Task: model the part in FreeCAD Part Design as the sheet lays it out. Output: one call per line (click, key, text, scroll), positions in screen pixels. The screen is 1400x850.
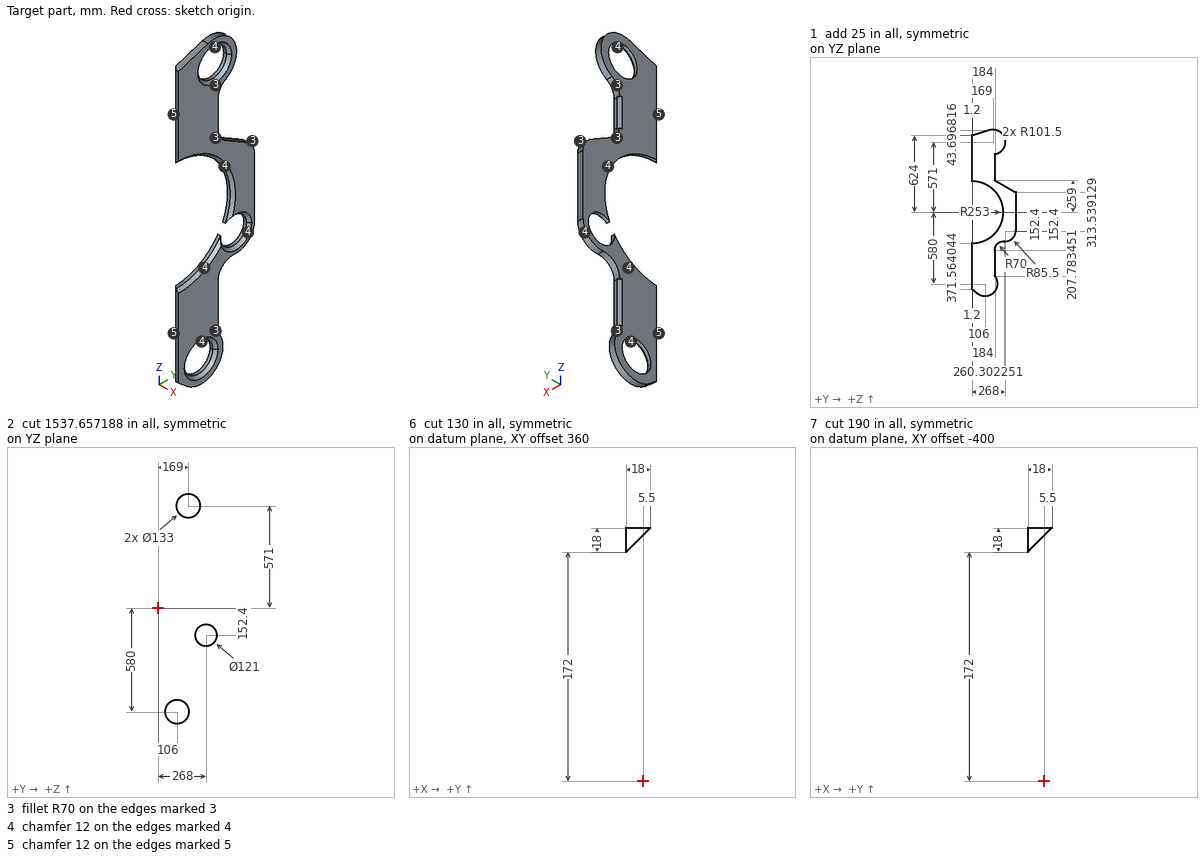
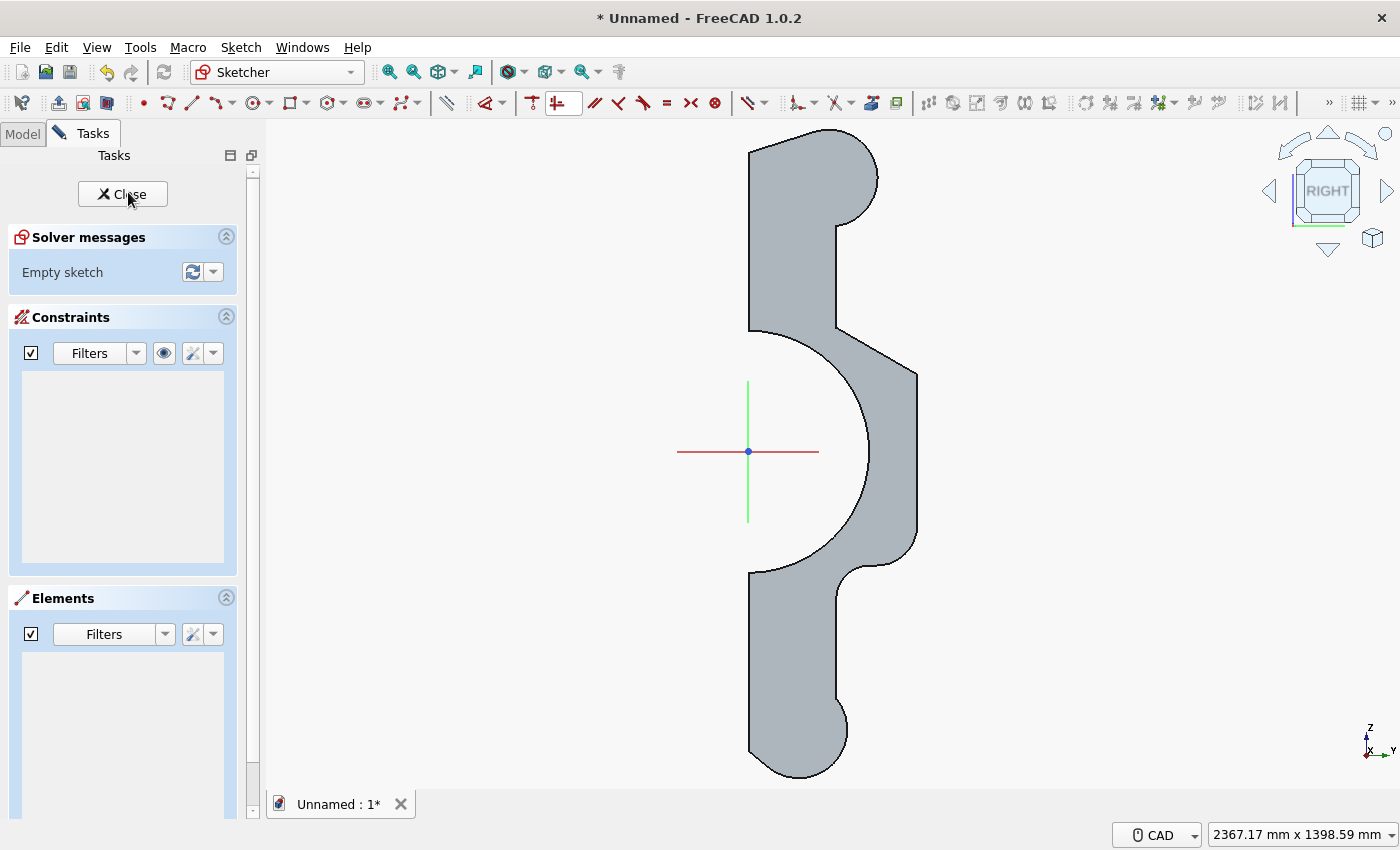
key(q)
key(s)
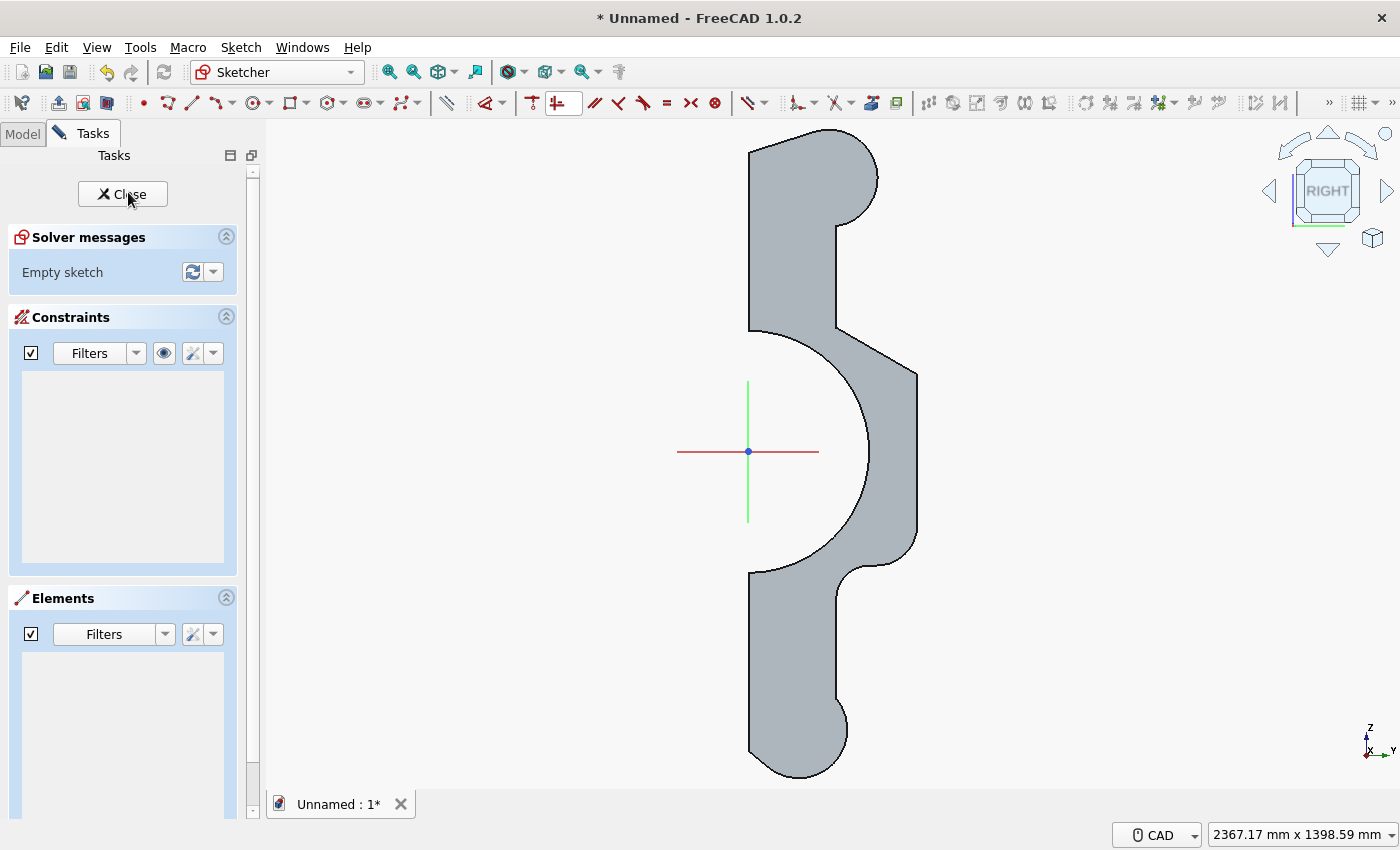
scroll(638, 454, down, 2)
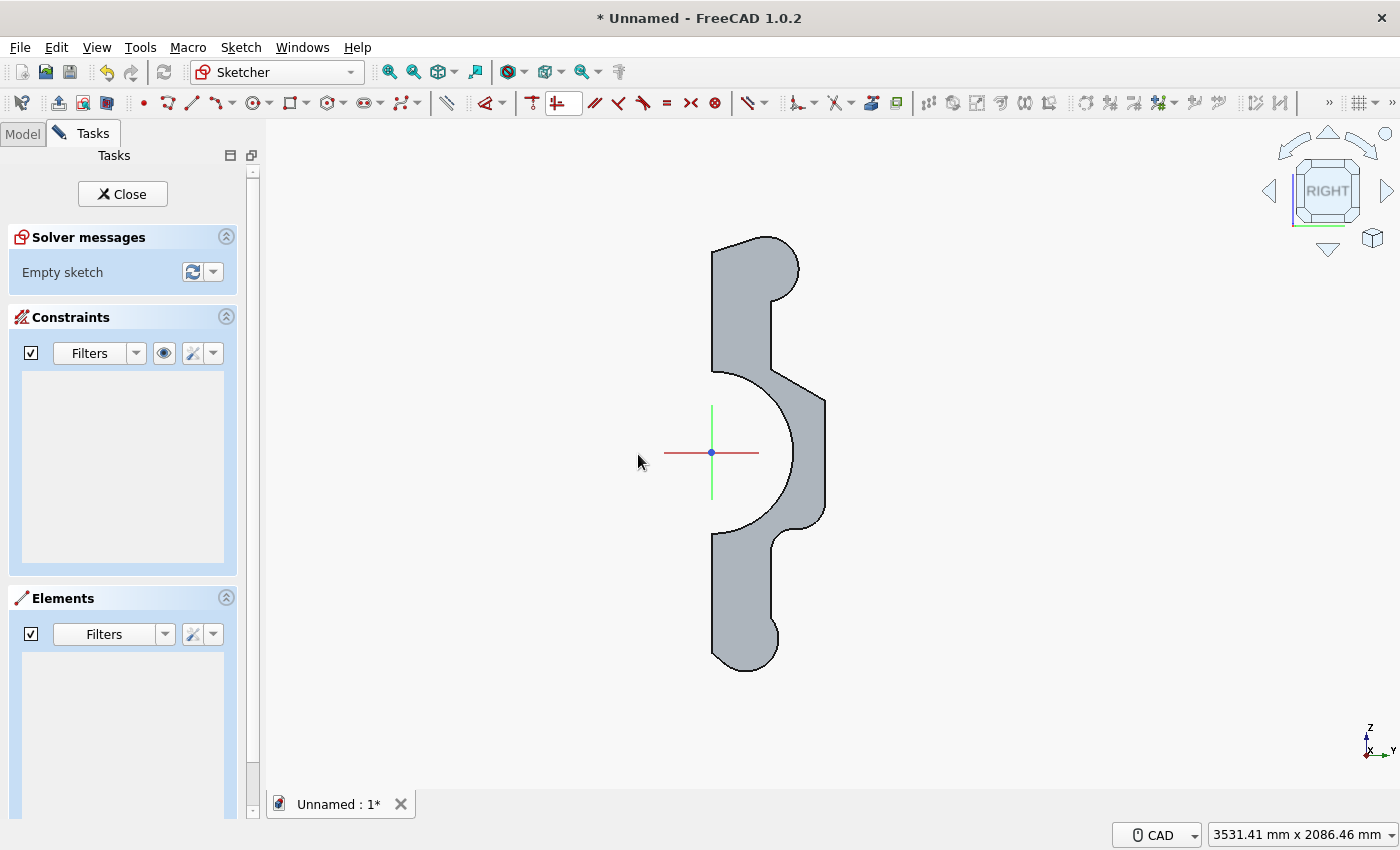
click(254, 104)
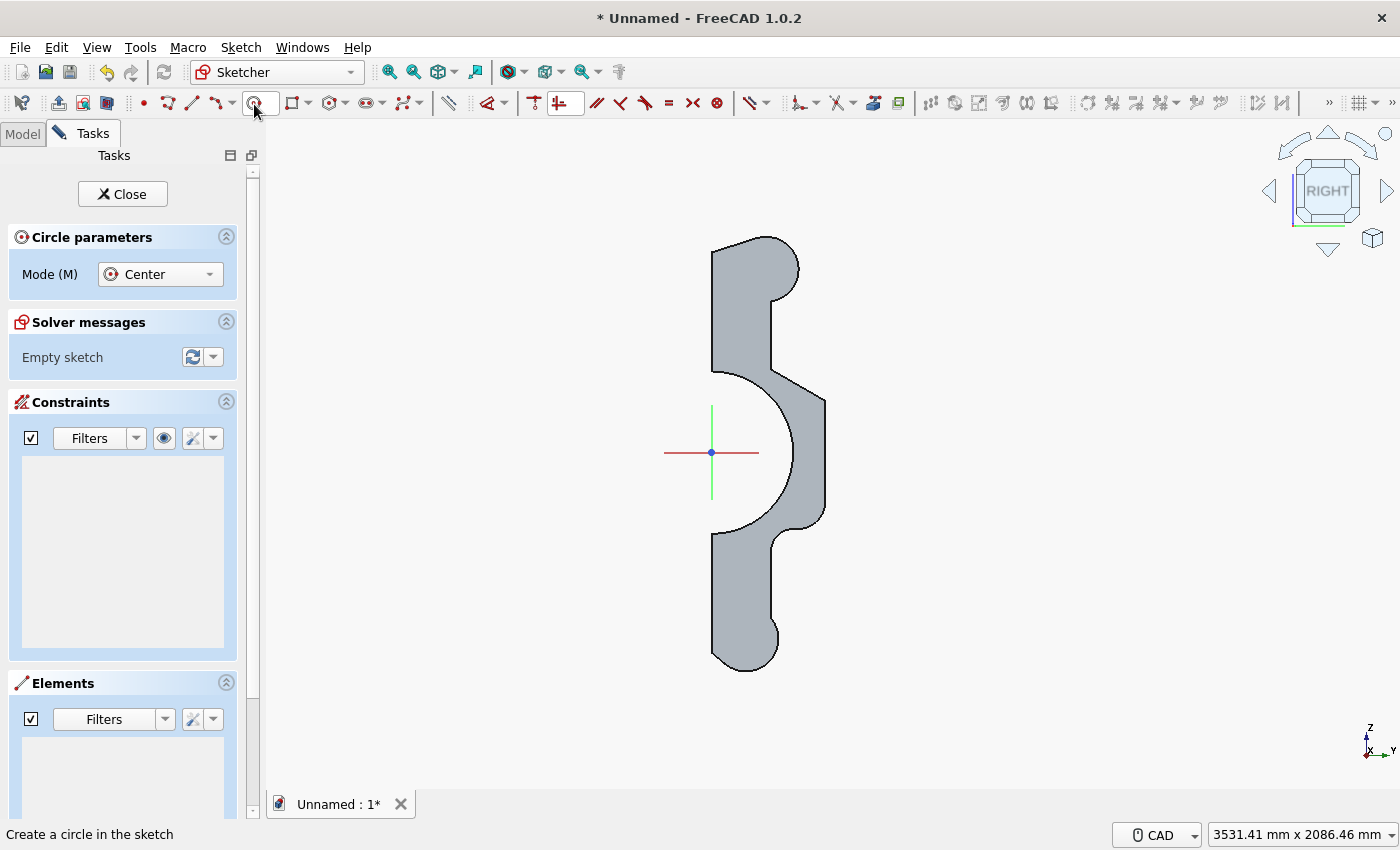
click(798, 502)
move(812, 488)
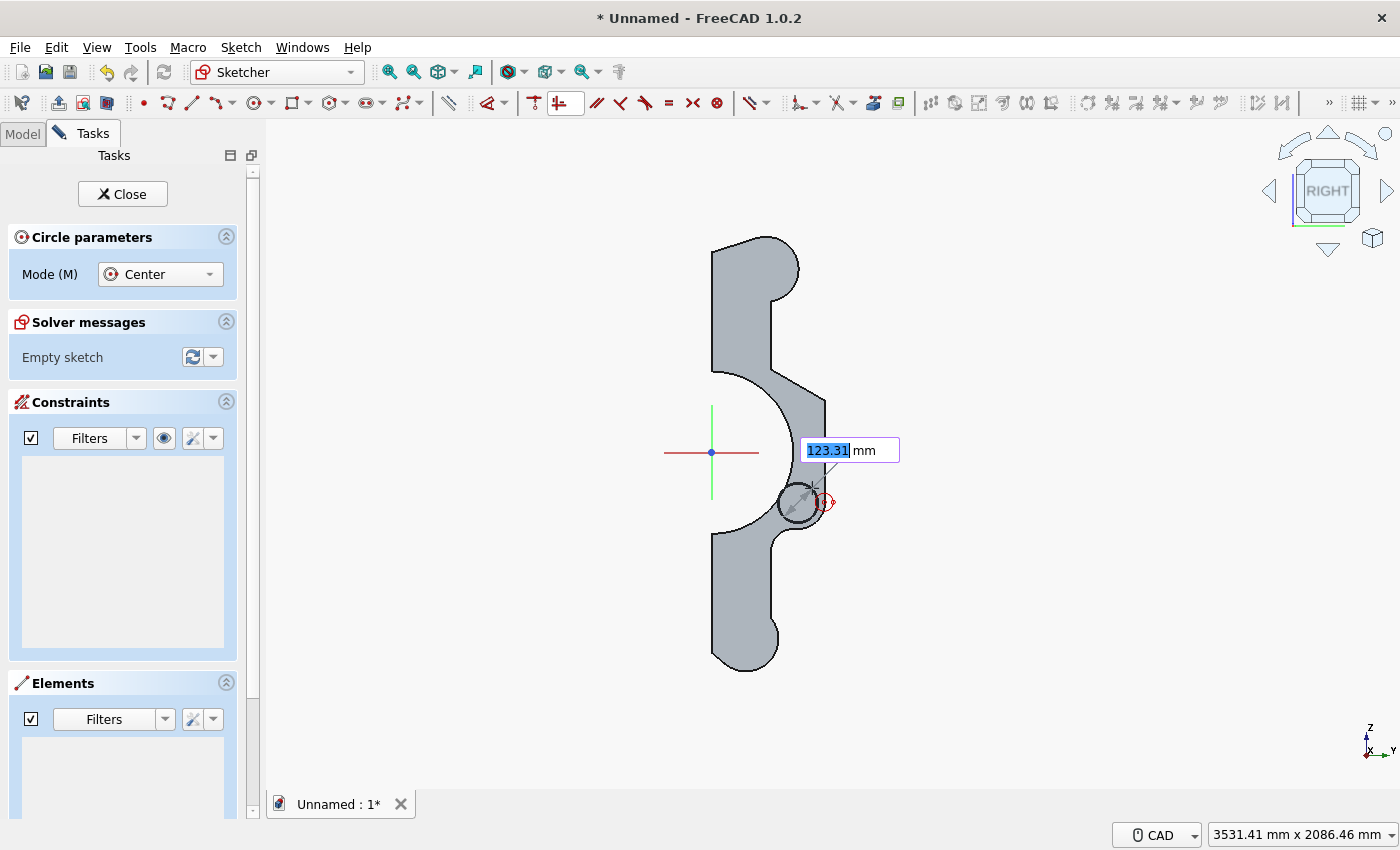
text(121)
key(Return)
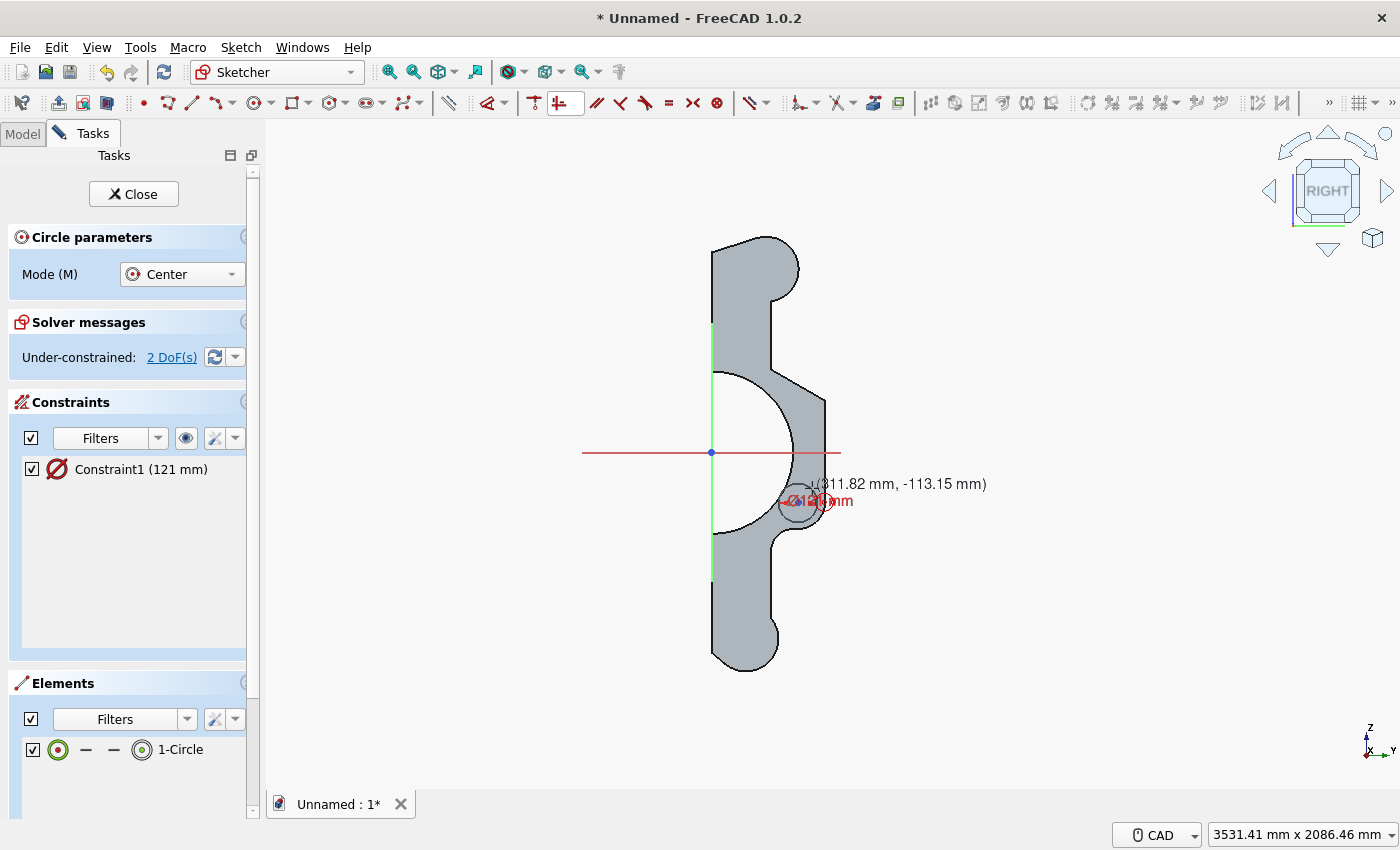
click(766, 269)
move(781, 254)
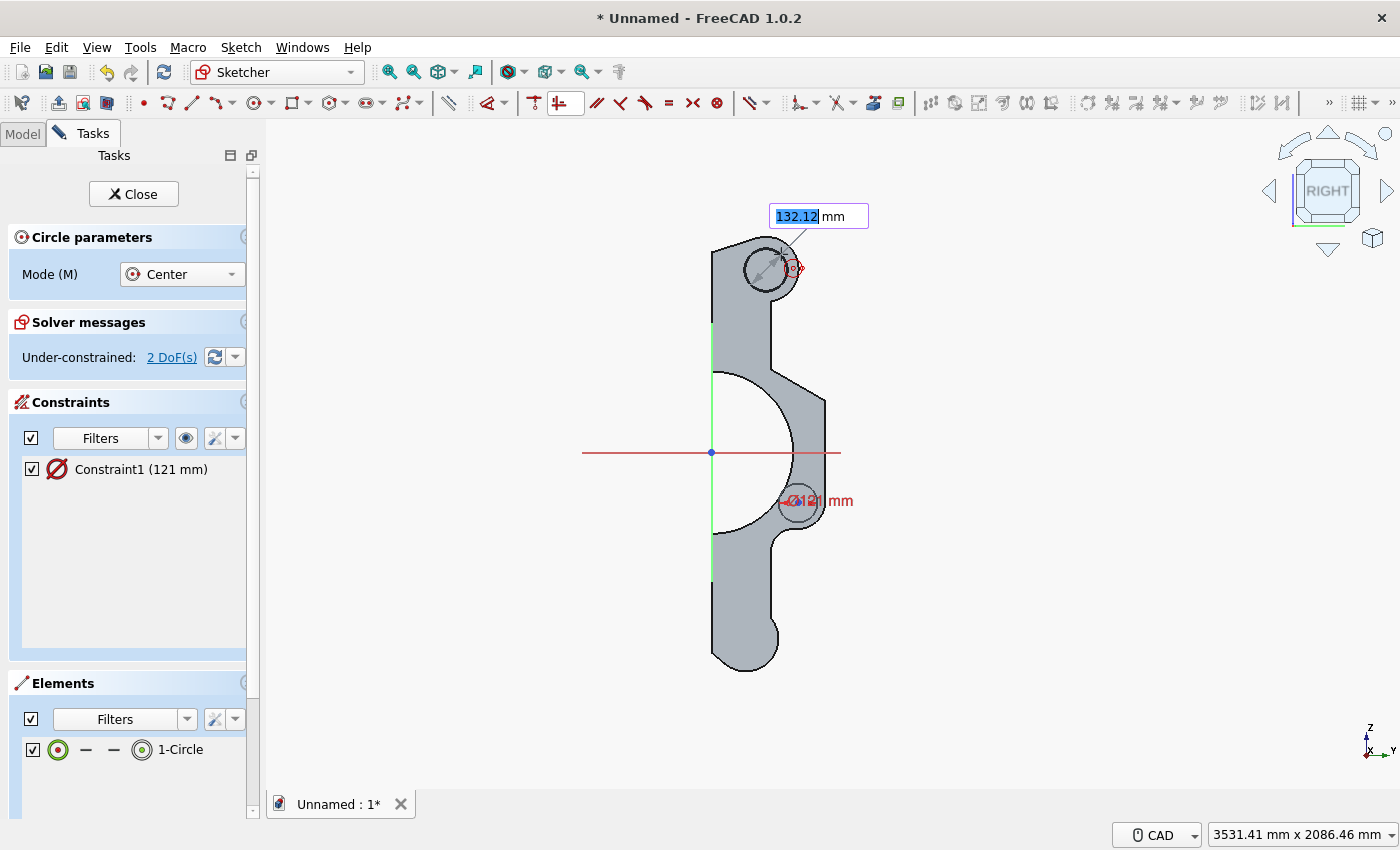
text(133)
key(Return)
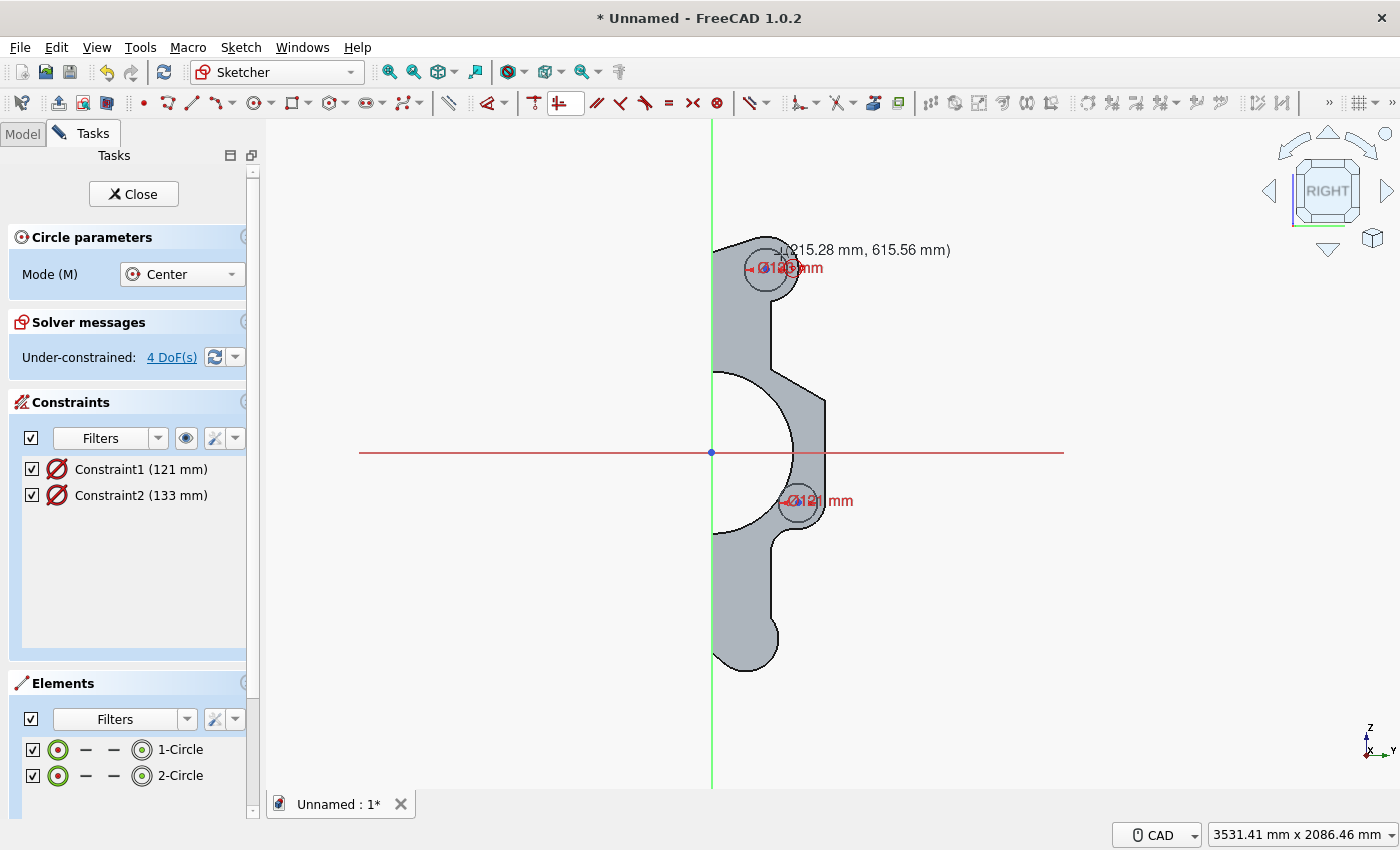
click(746, 639)
move(761, 624)